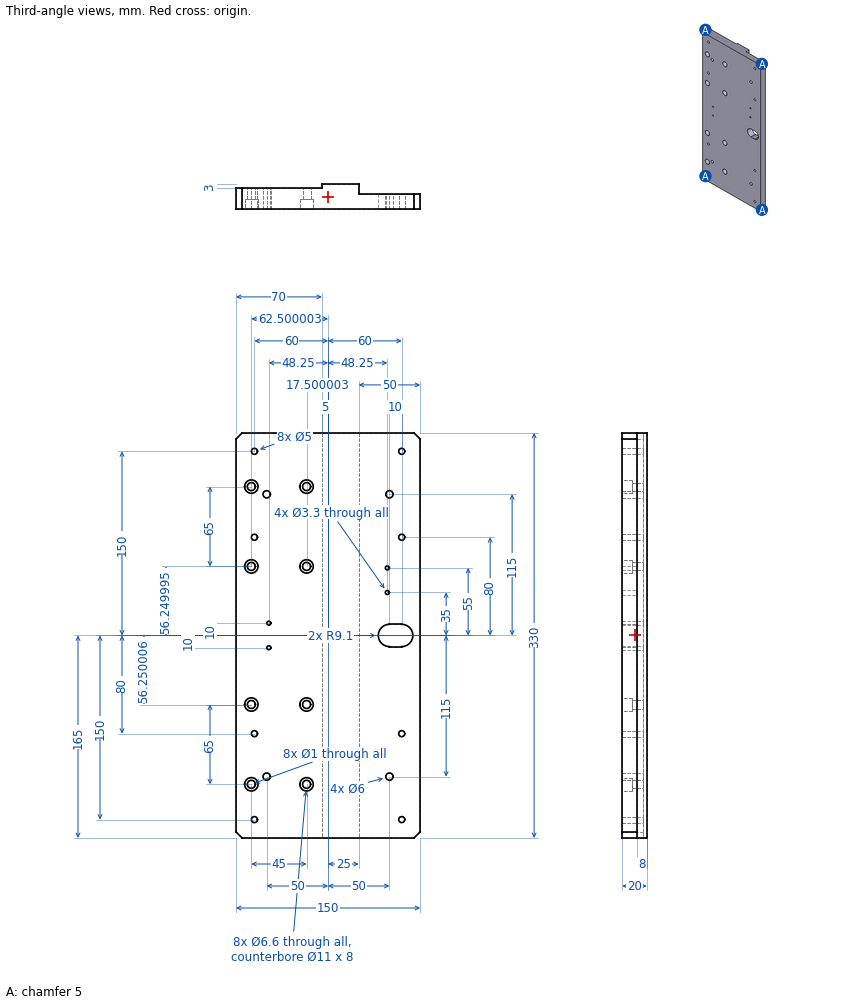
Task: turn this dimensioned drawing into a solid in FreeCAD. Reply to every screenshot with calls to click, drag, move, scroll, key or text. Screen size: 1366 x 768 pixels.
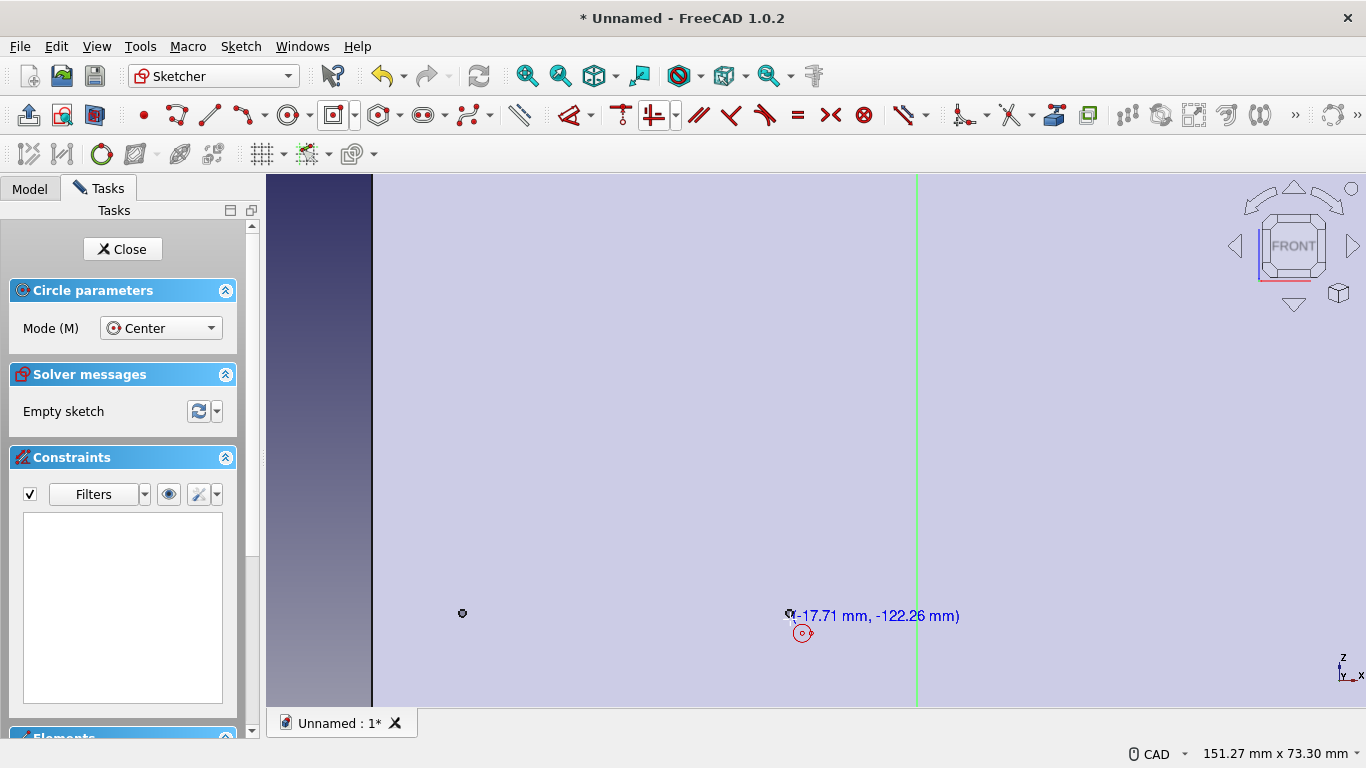
scroll(765, 620, down, 8)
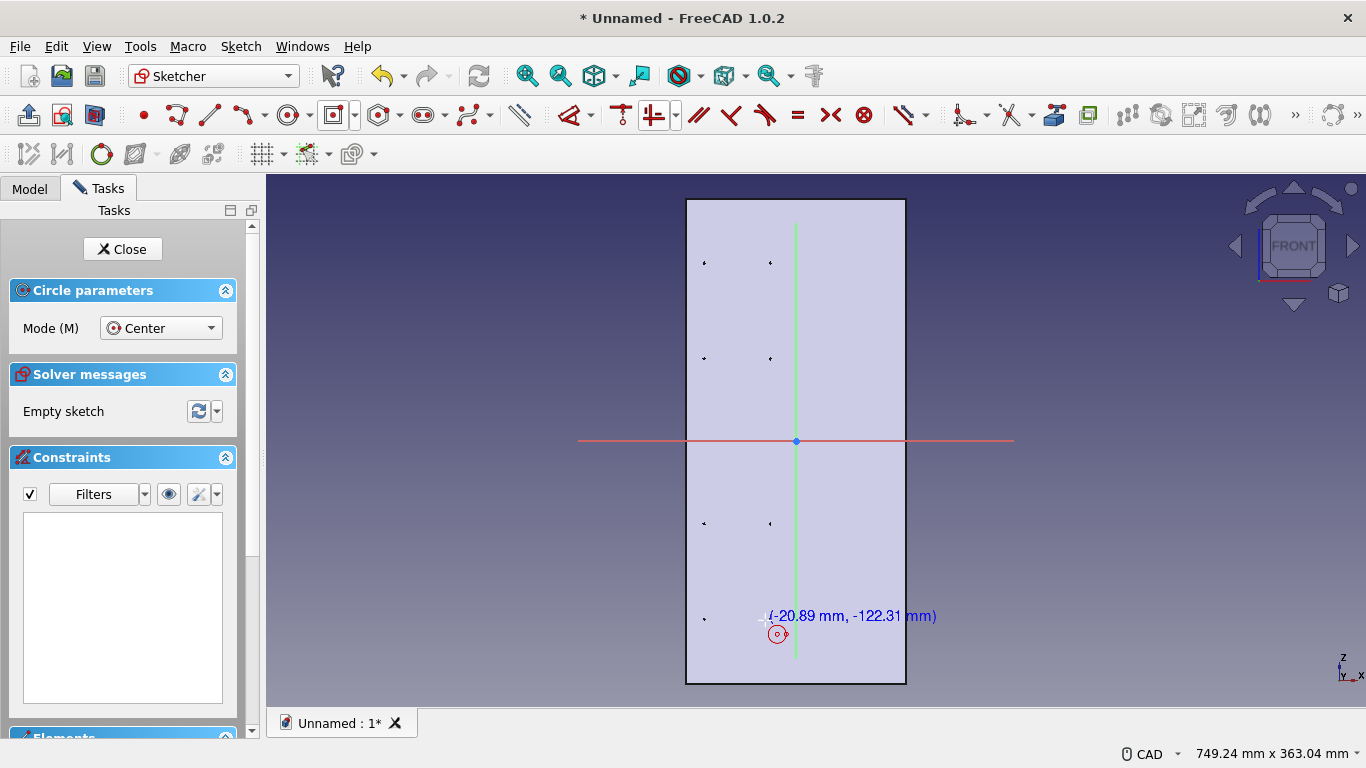
click(770, 619)
move(774, 616)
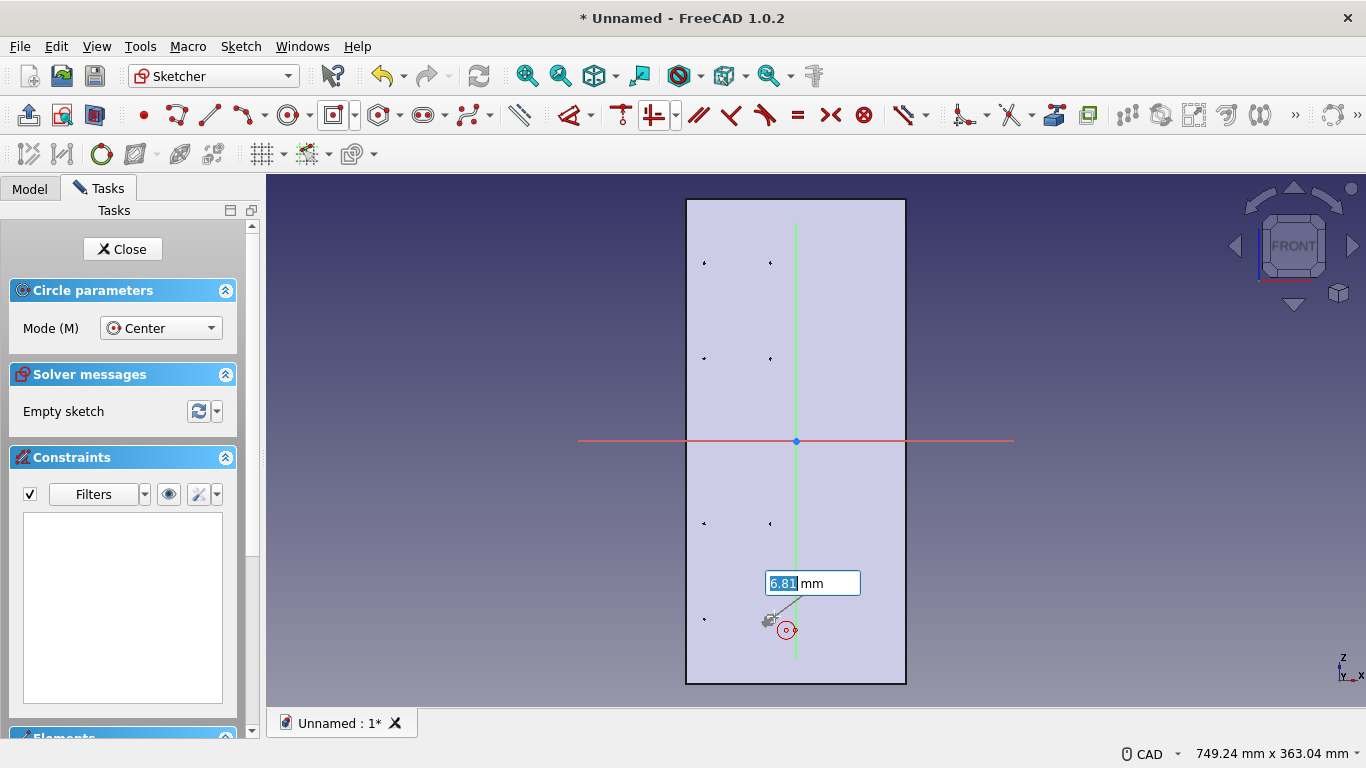
text(6.6)
key(Return)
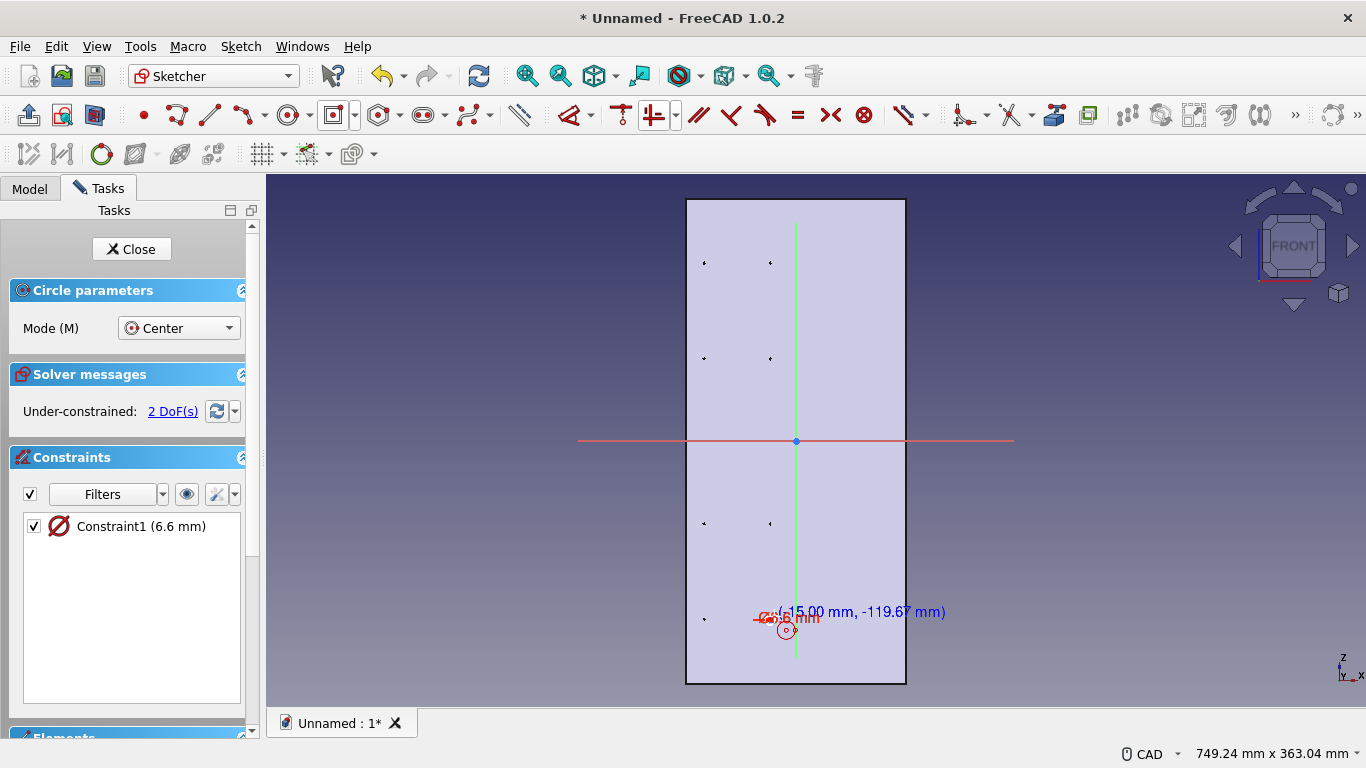
scroll(704, 619, up, 8)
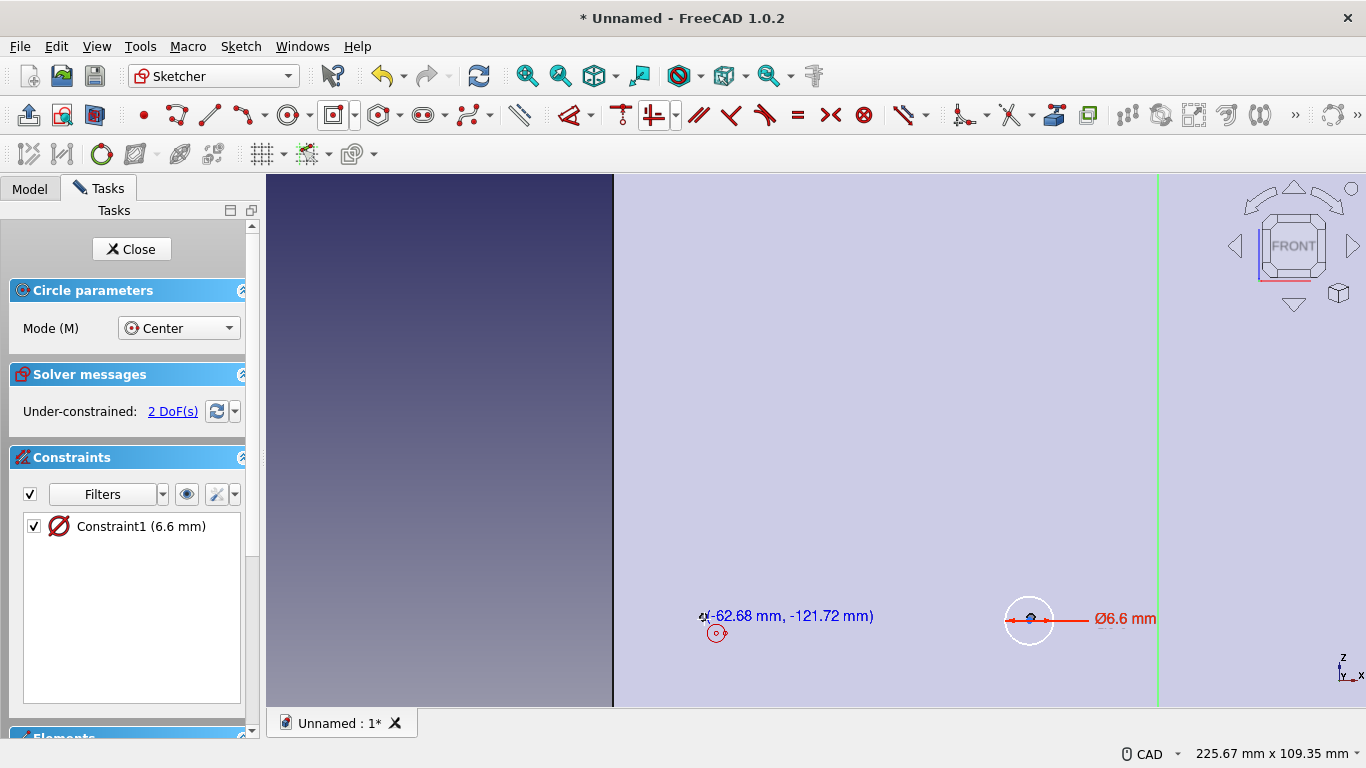
scroll(704, 619, down, 8)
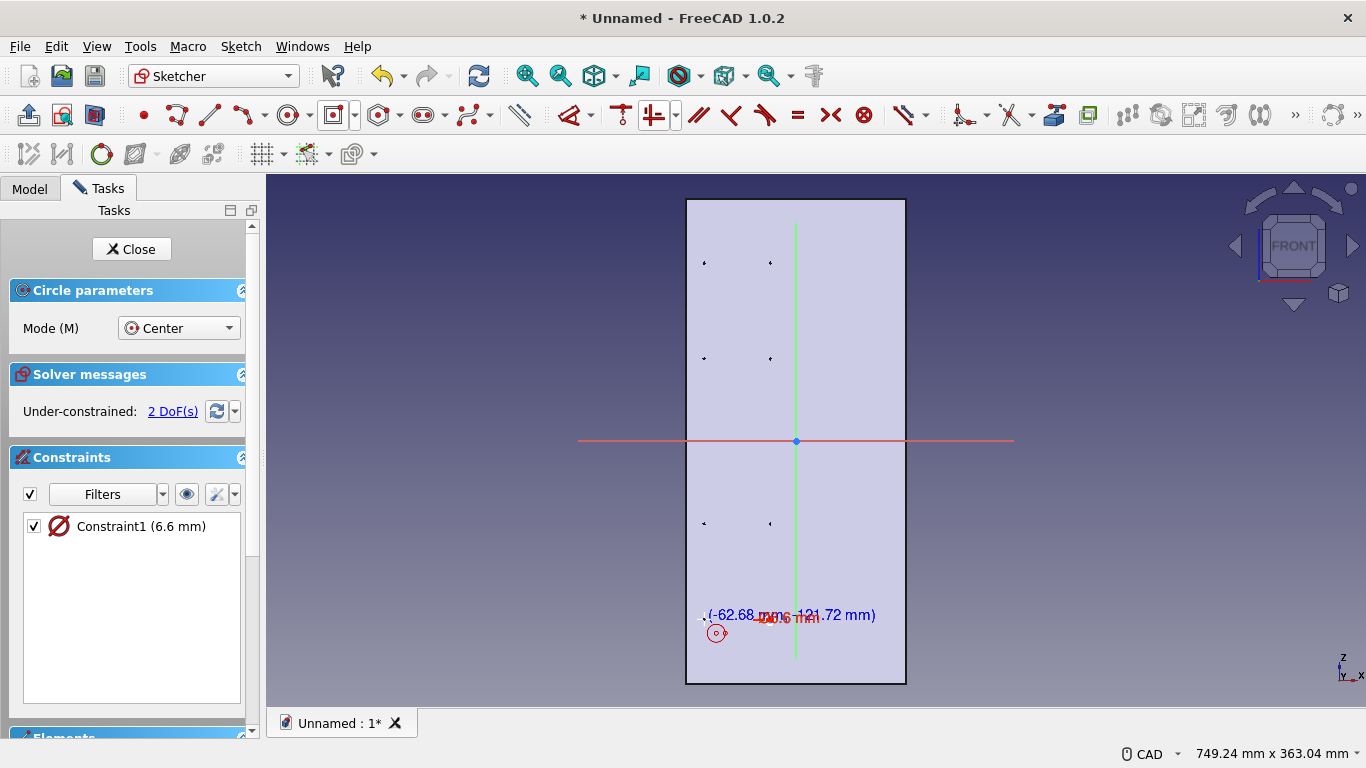
click(704, 619)
move(708, 616)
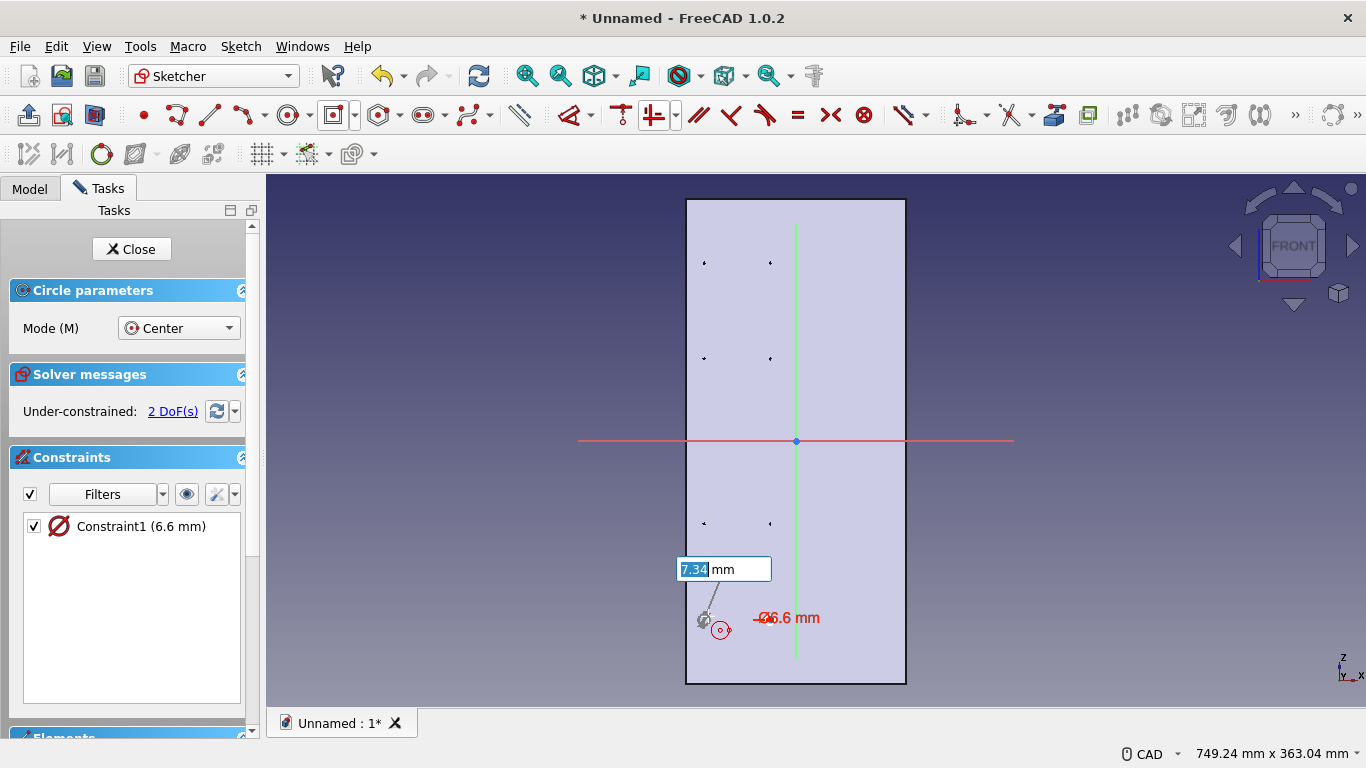
text(6.6)
key(Return)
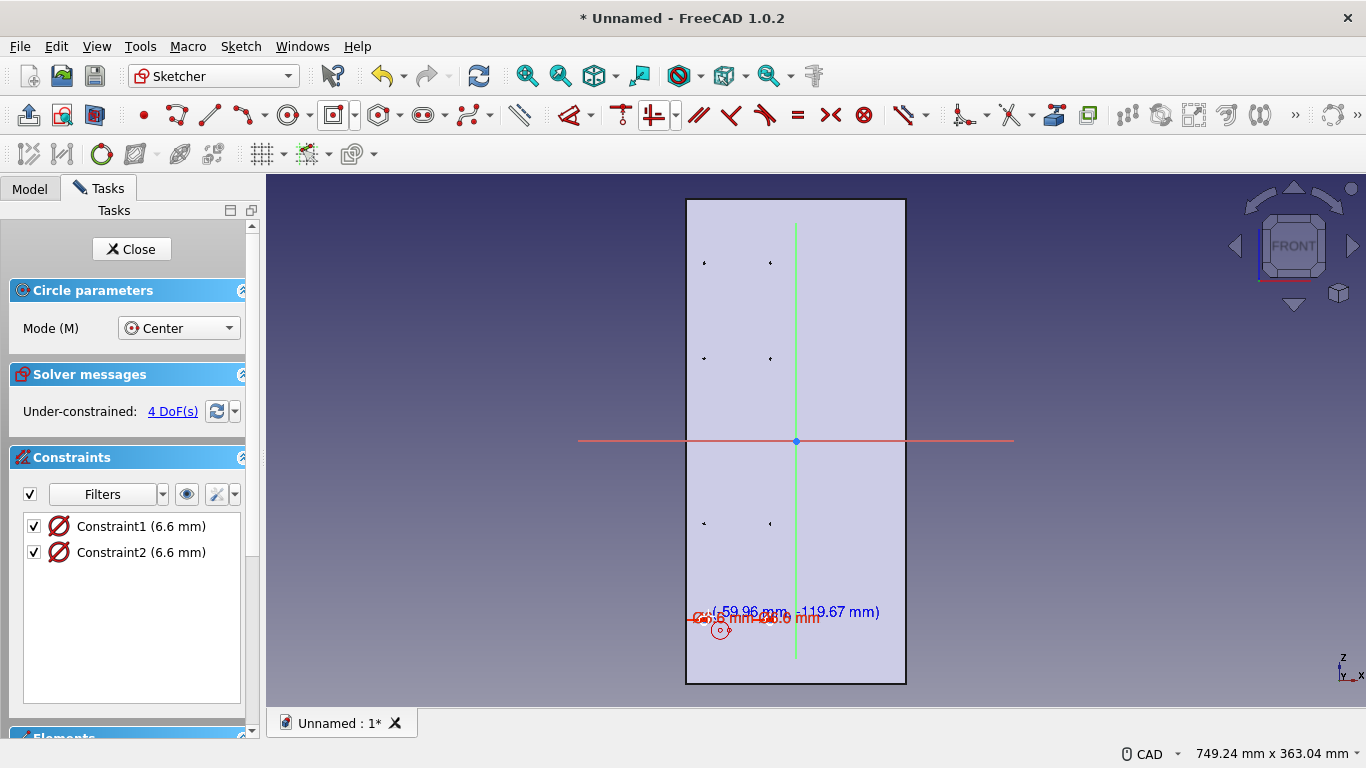
scroll(770, 524, up, 8)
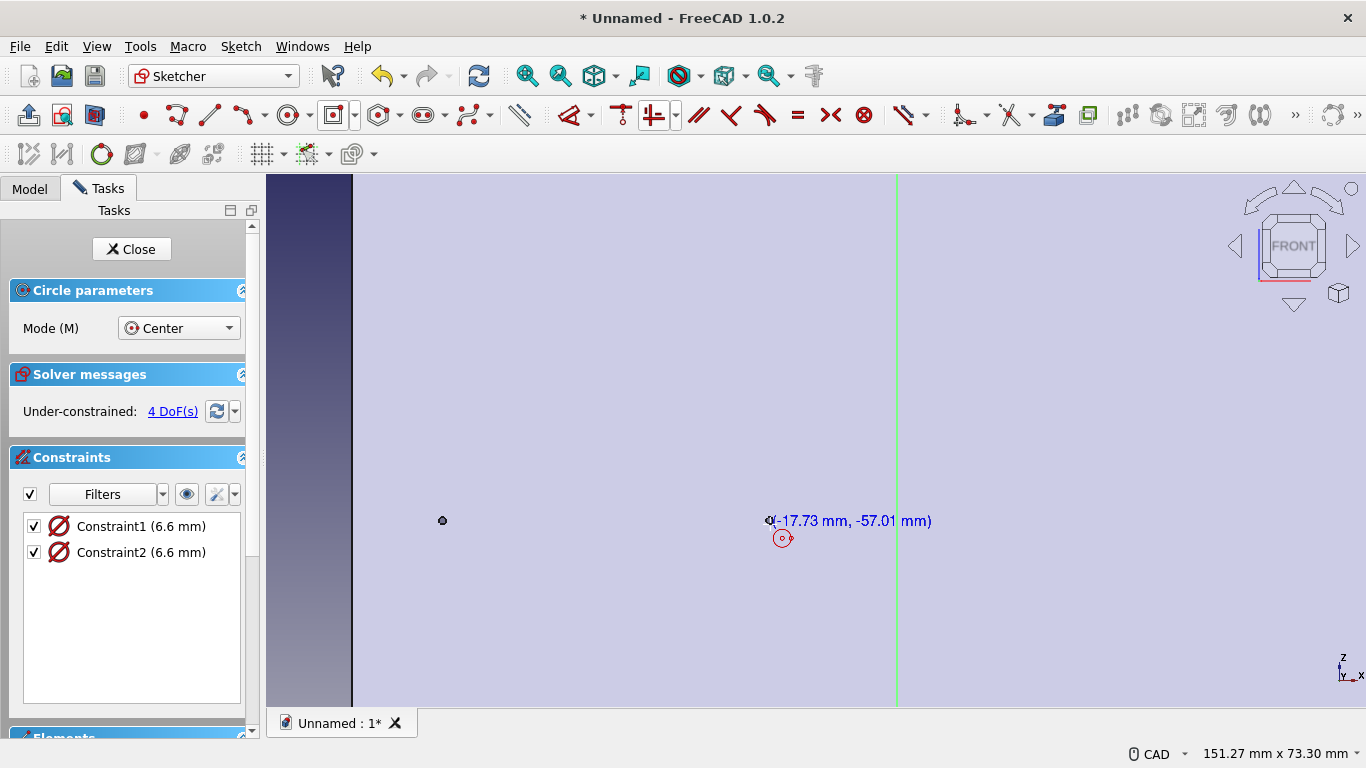
scroll(770, 524, down, 8)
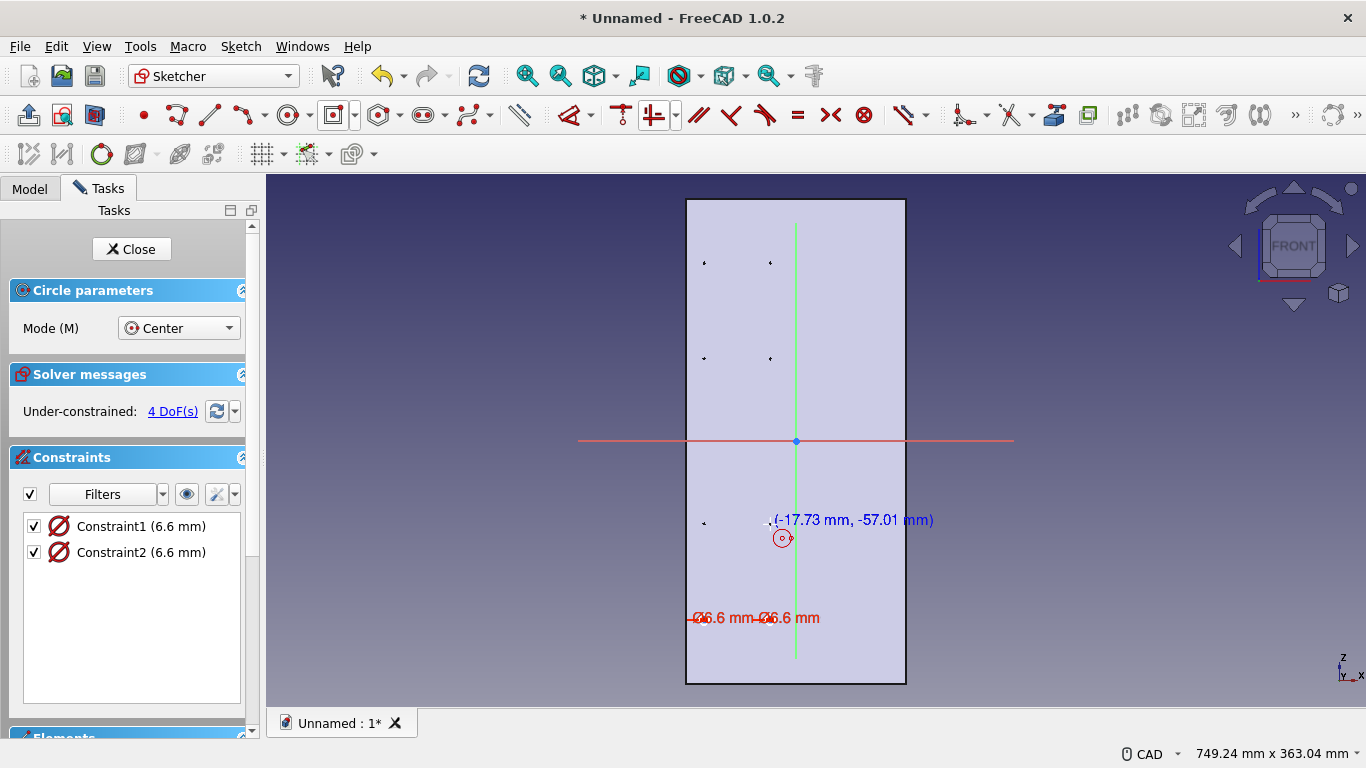
click(770, 524)
move(774, 520)